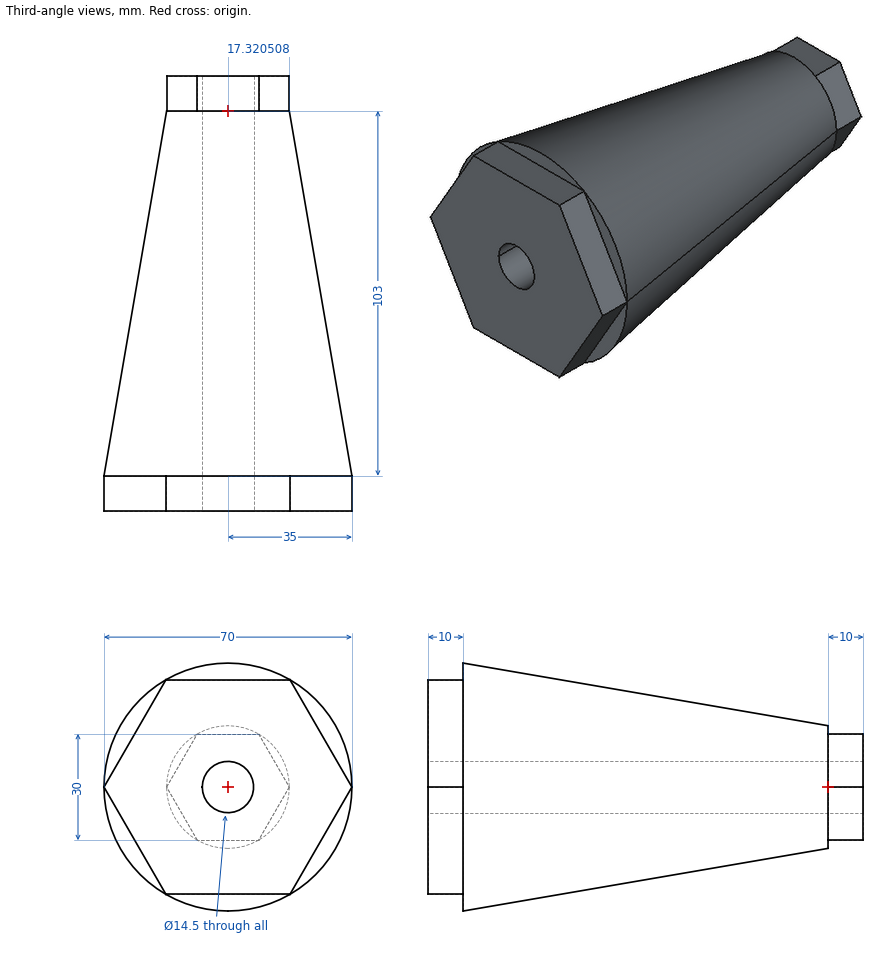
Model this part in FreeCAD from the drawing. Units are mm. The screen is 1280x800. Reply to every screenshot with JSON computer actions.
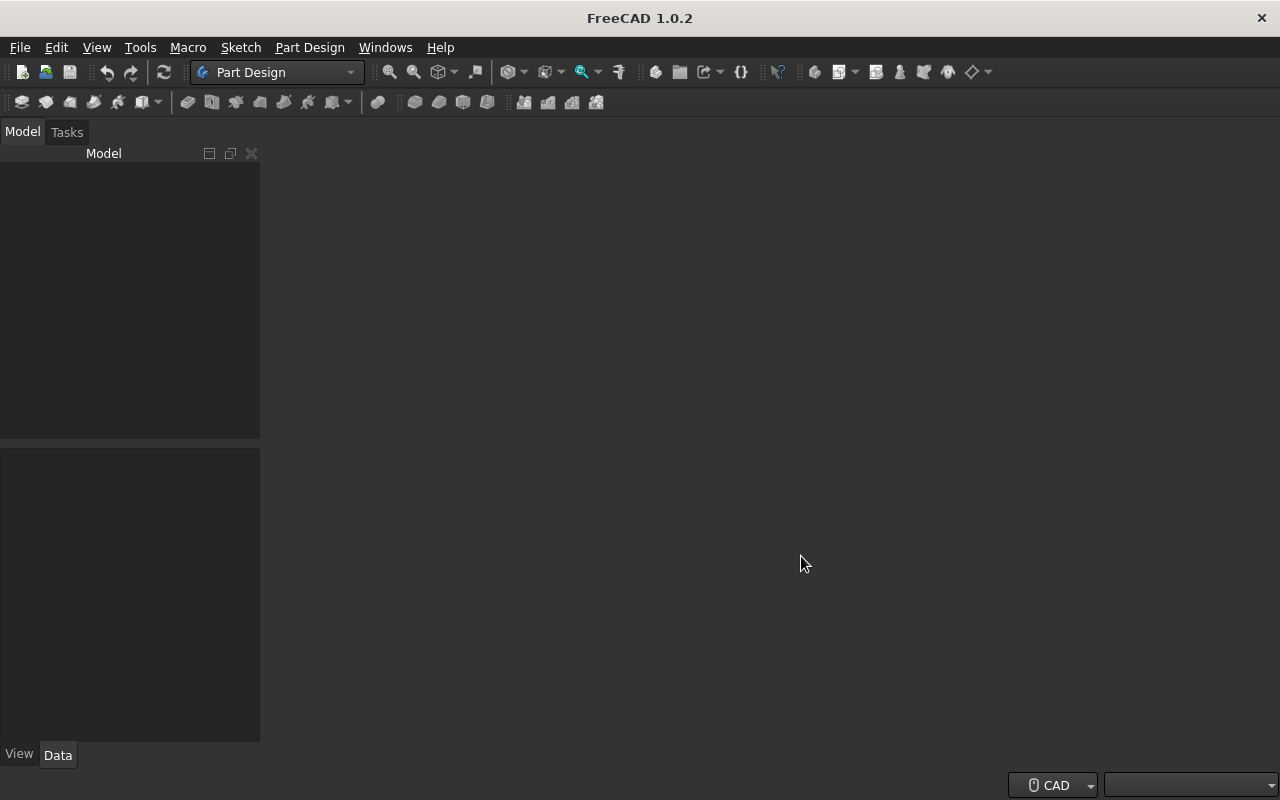
{"action": "left_click", "coordinate": [22, 72]}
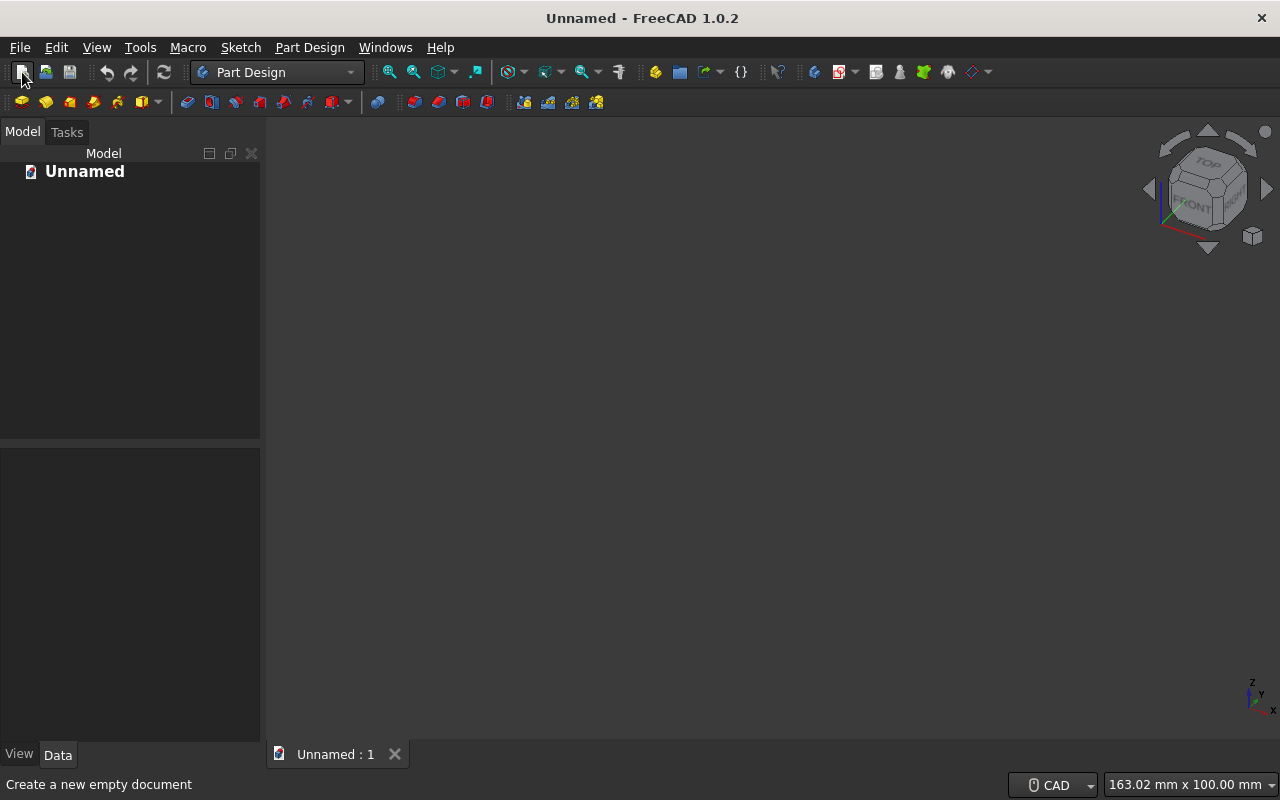
{"action": "left_click", "coordinate": [840, 72]}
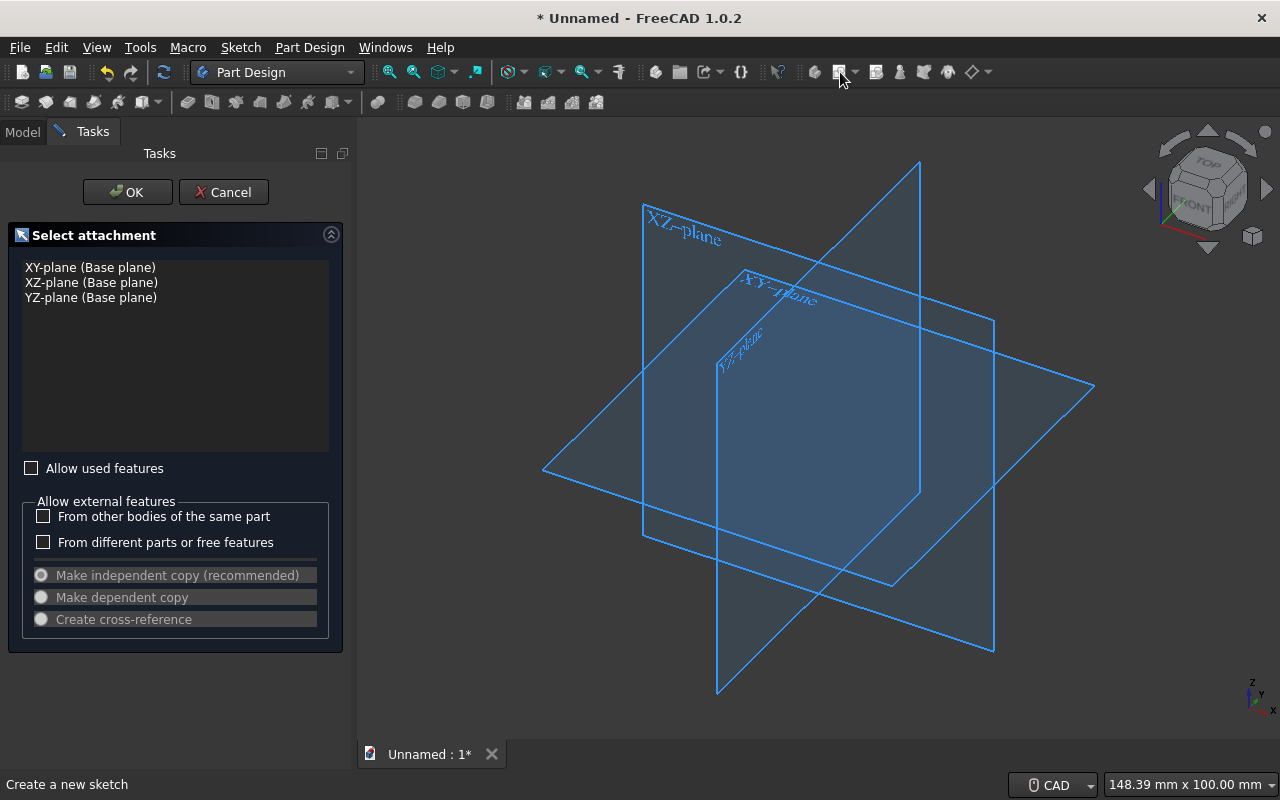
{"action": "left_click", "coordinate": [82, 282]}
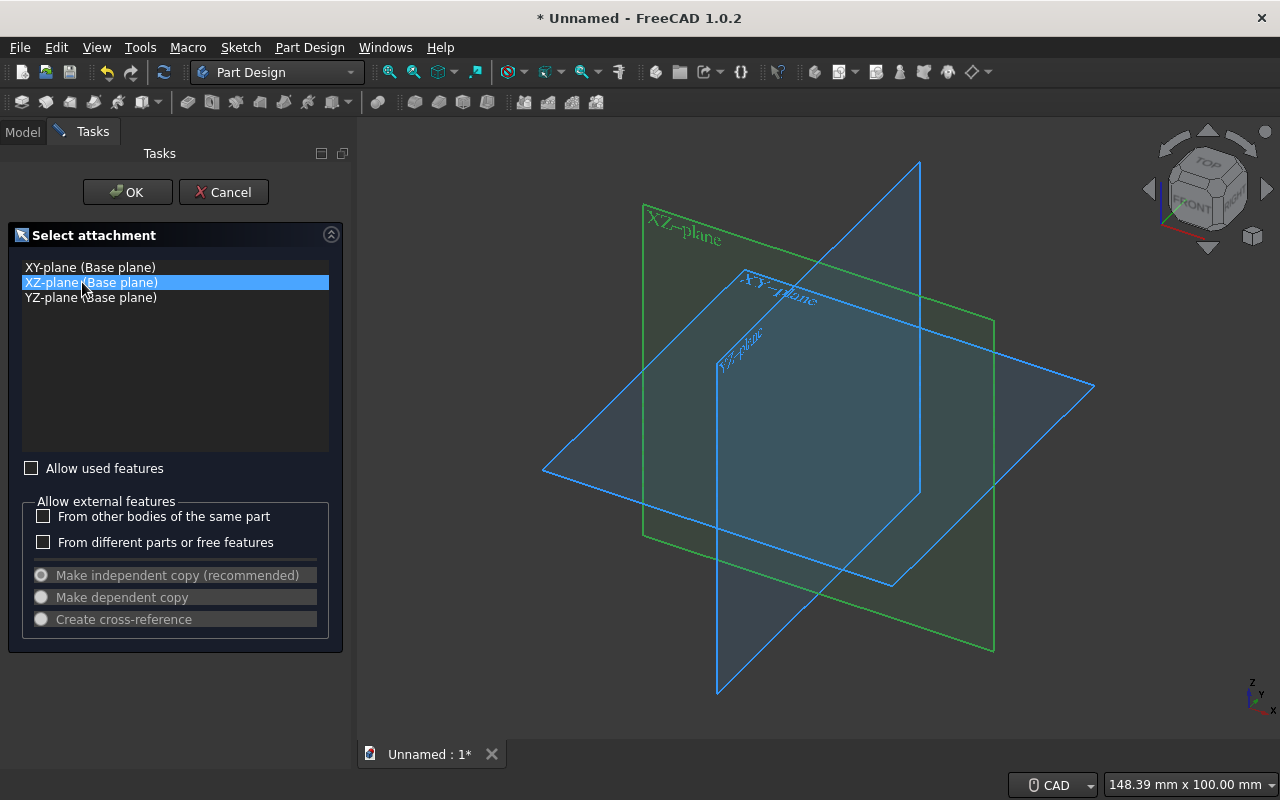
{"action": "left_click", "coordinate": [128, 192]}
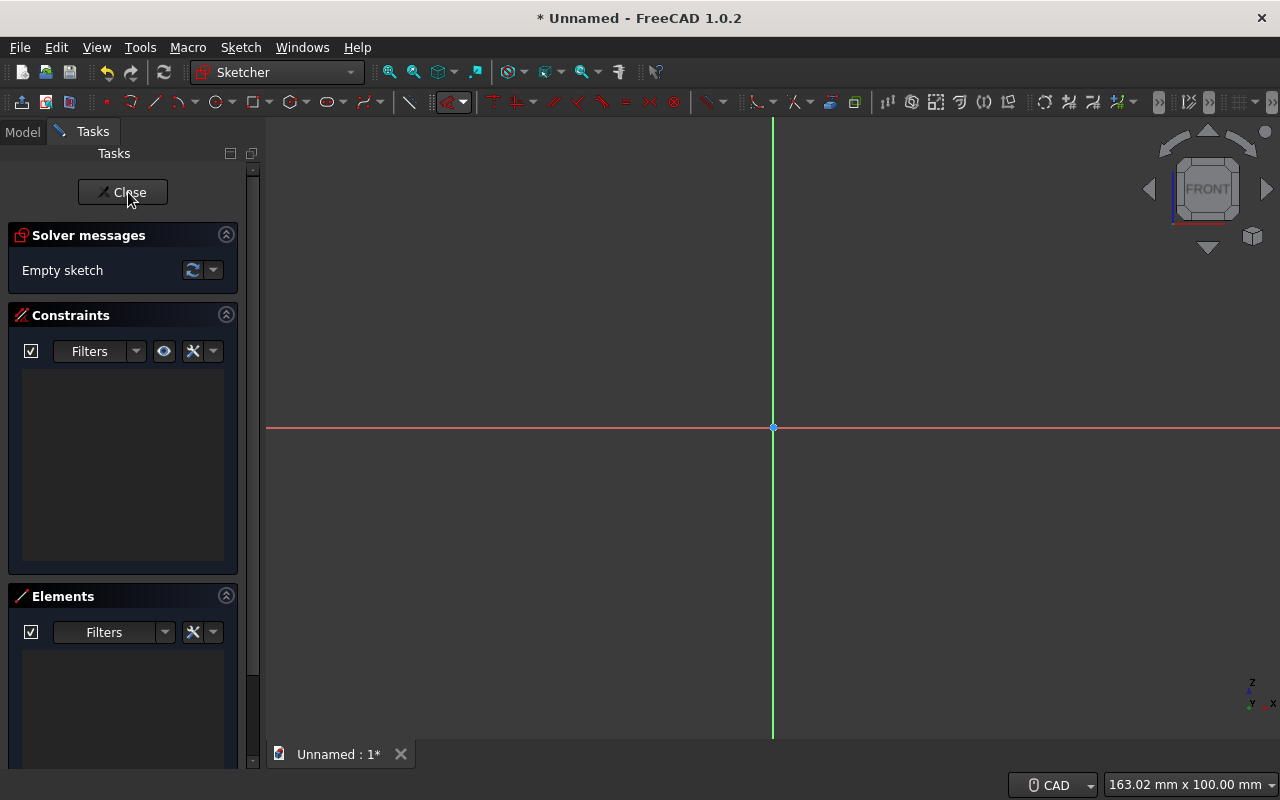
{"action": "scroll", "coordinate": [829, 428], "scroll_direction": "up", "scroll_amount": 4}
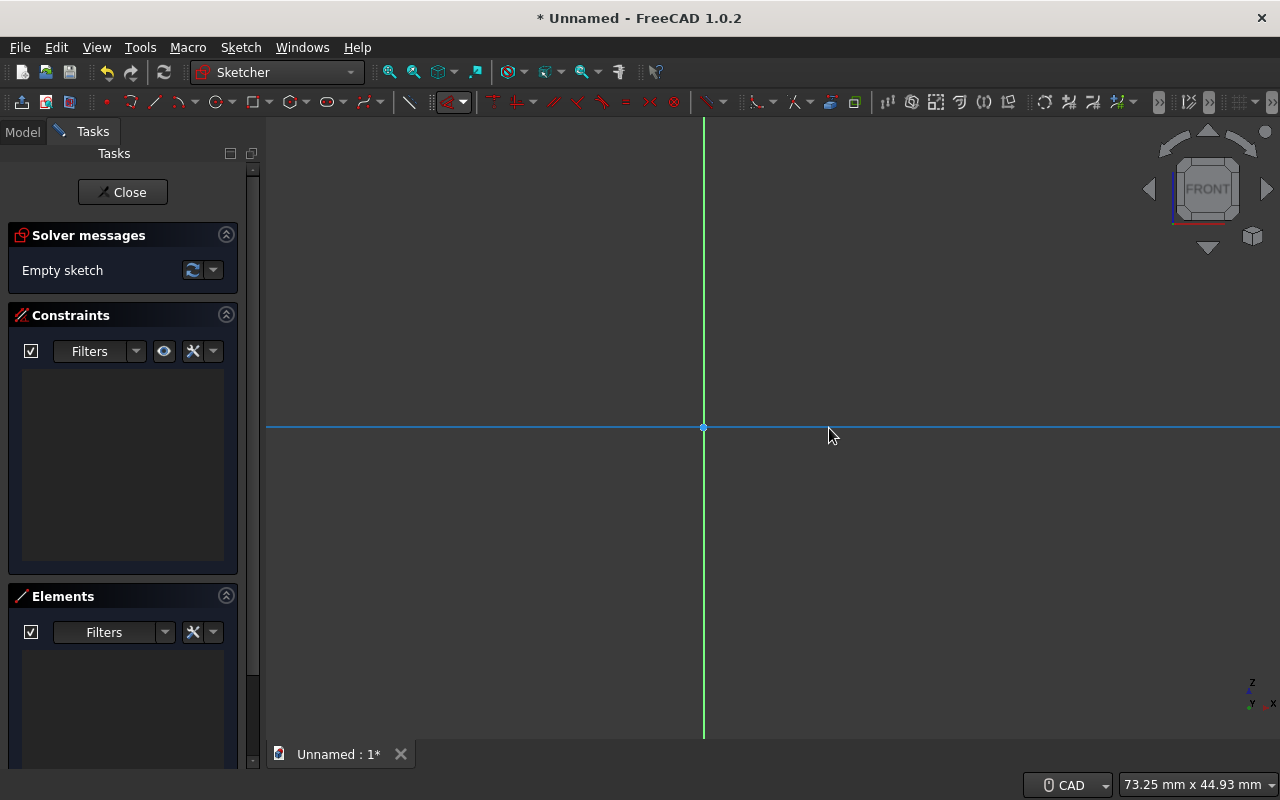
{"action": "left_click", "coordinate": [290, 102]}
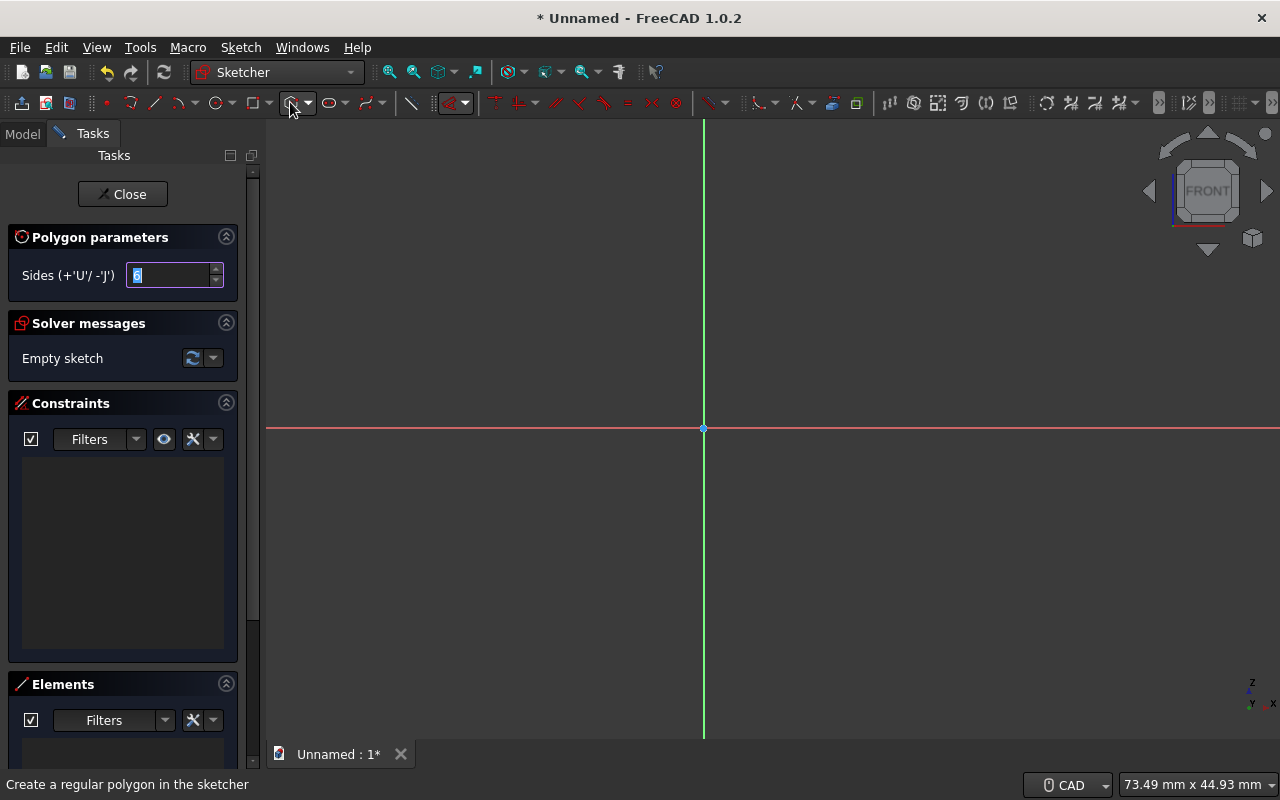
{"action": "left_click", "coordinate": [704, 428]}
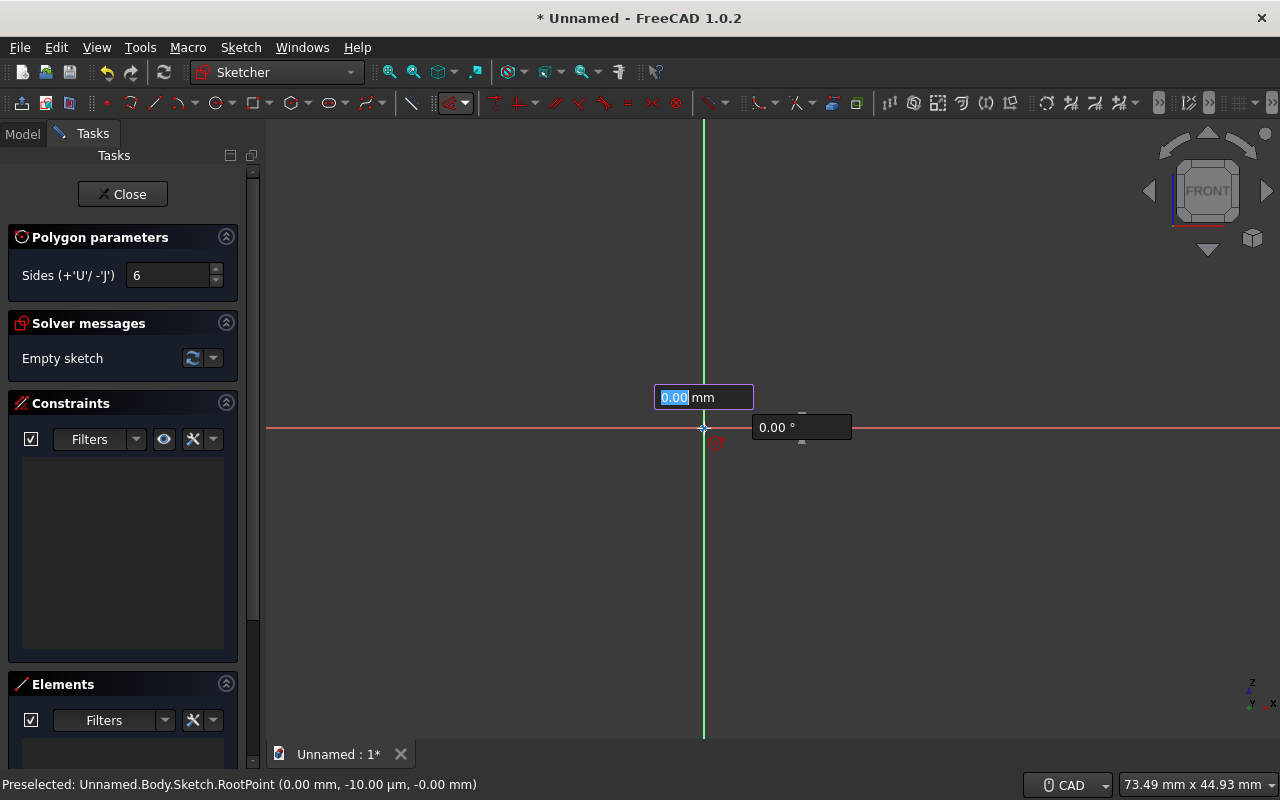
{"action": "left_click", "coordinate": [943, 428]}
{"action": "right_click", "coordinate": [943, 428]}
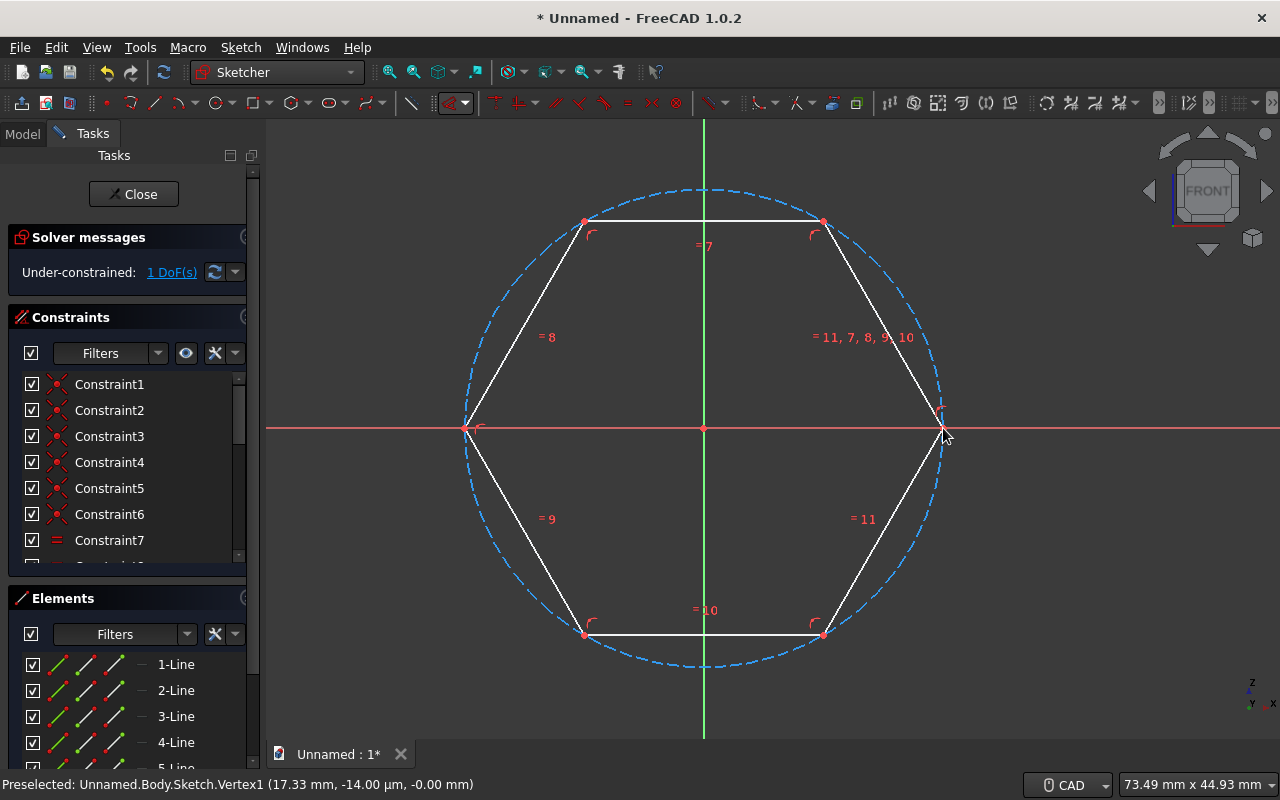
{"action": "left_click", "coordinate": [450, 104]}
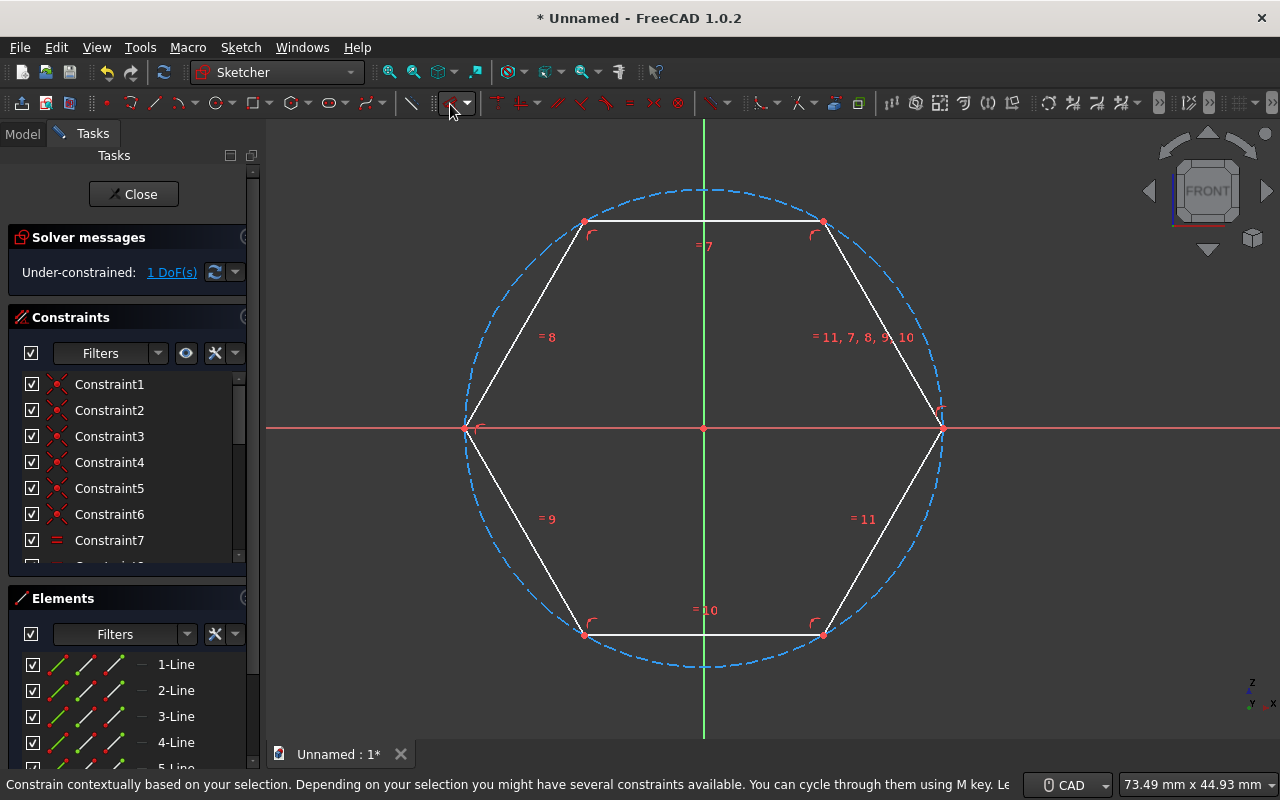
{"action": "left_click", "coordinate": [584, 635]}